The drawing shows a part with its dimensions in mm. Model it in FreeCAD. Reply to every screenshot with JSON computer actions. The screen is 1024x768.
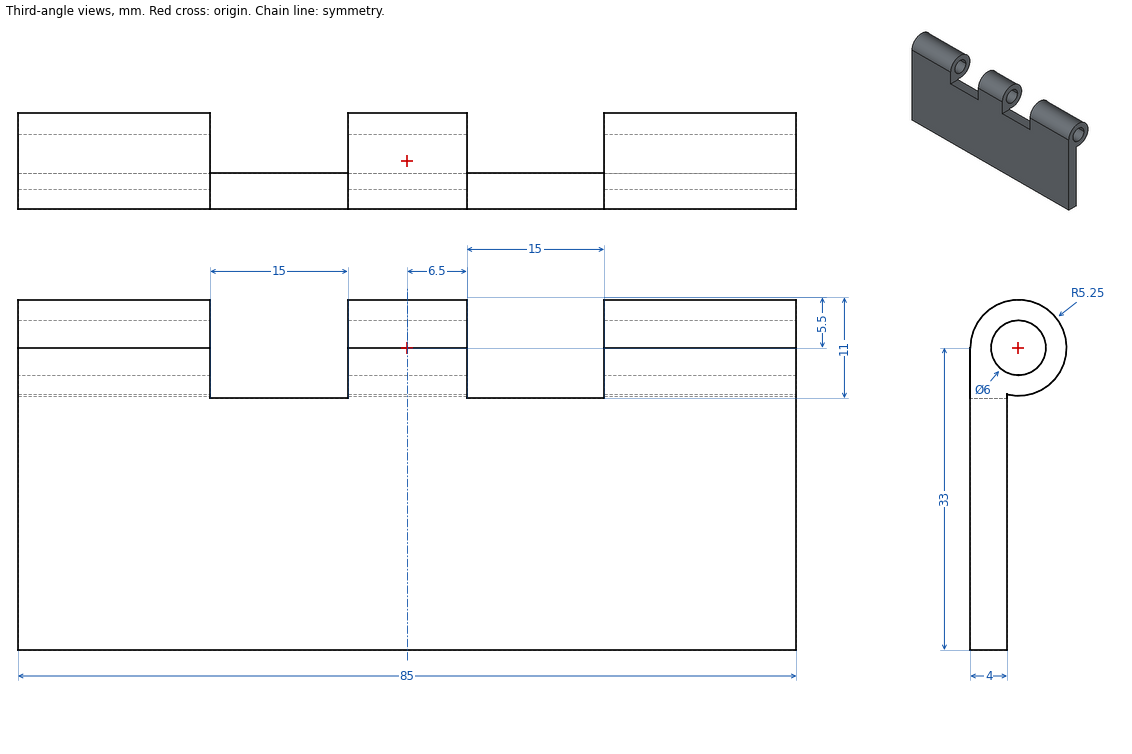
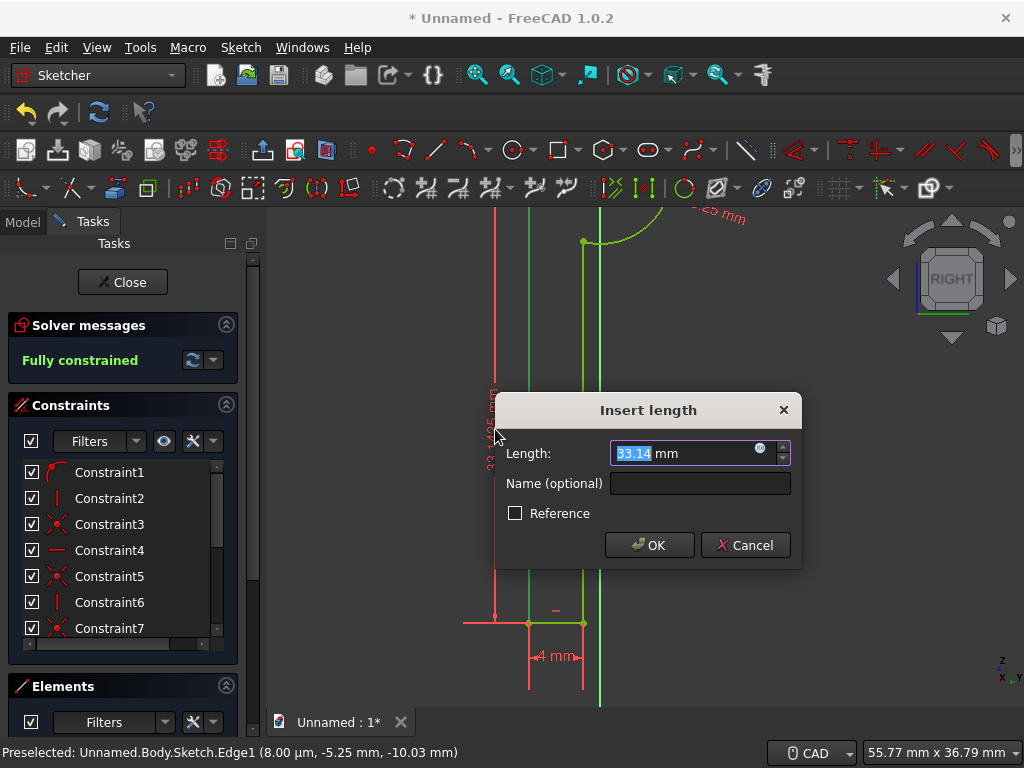
{"action": "type", "text": "33"}
{"action": "key", "text": "Return"}
{"action": "key", "text": "Escape"}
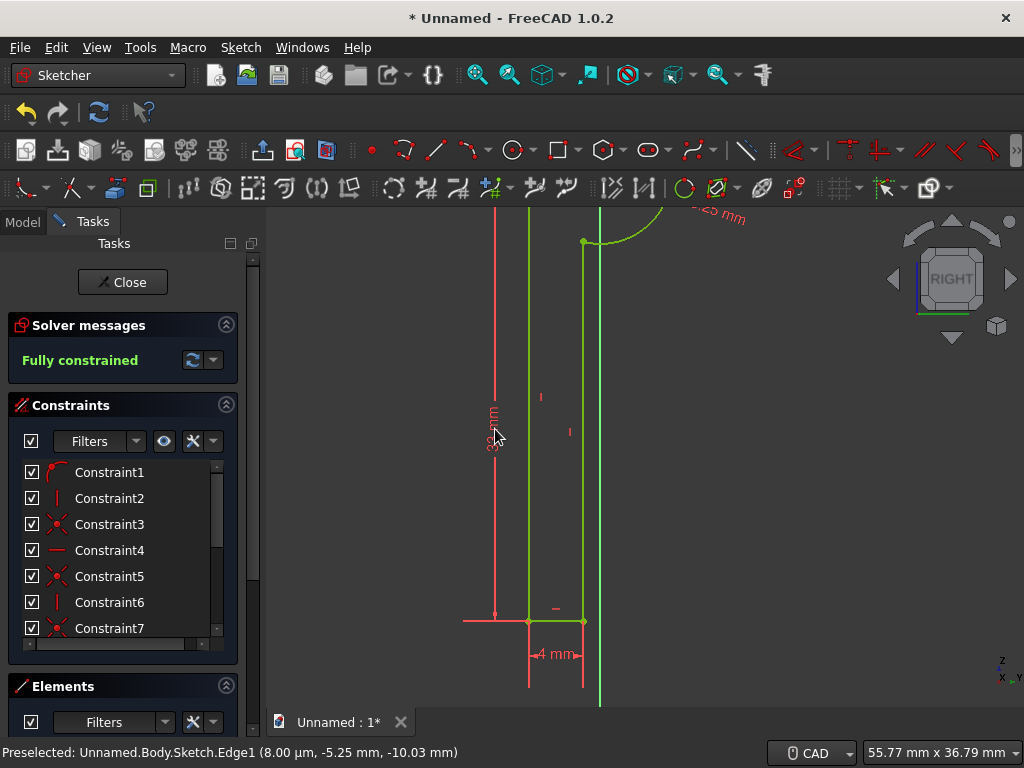
{"action": "left_click", "coordinate": [123, 282]}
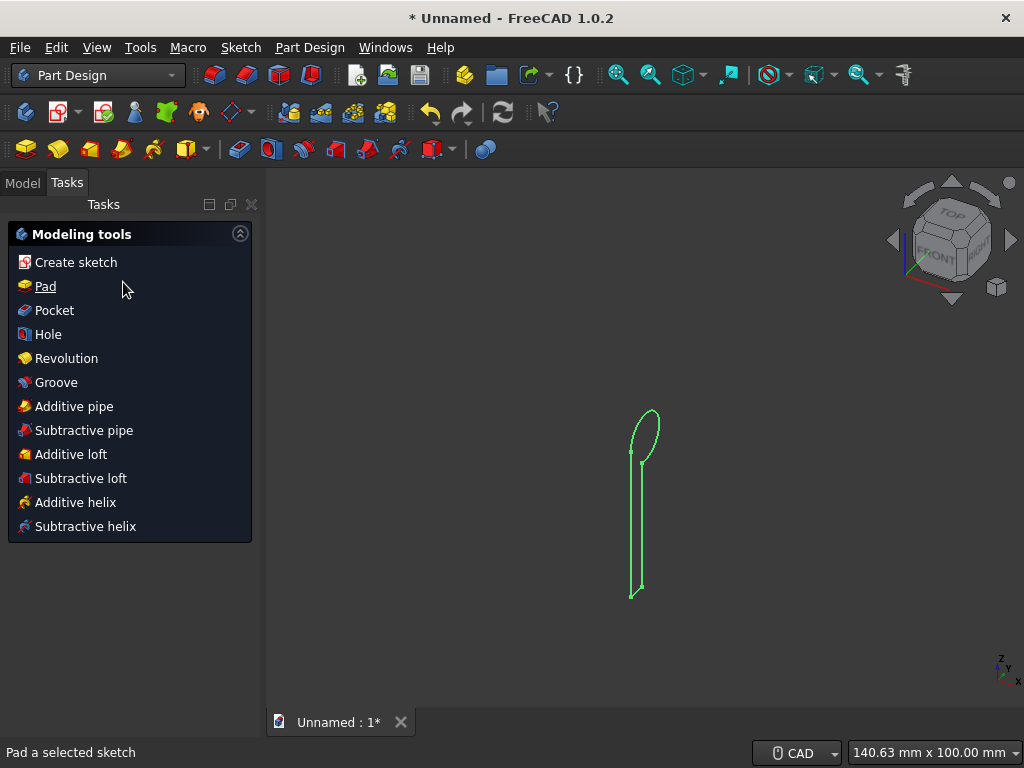
{"action": "left_click", "coordinate": [26, 150]}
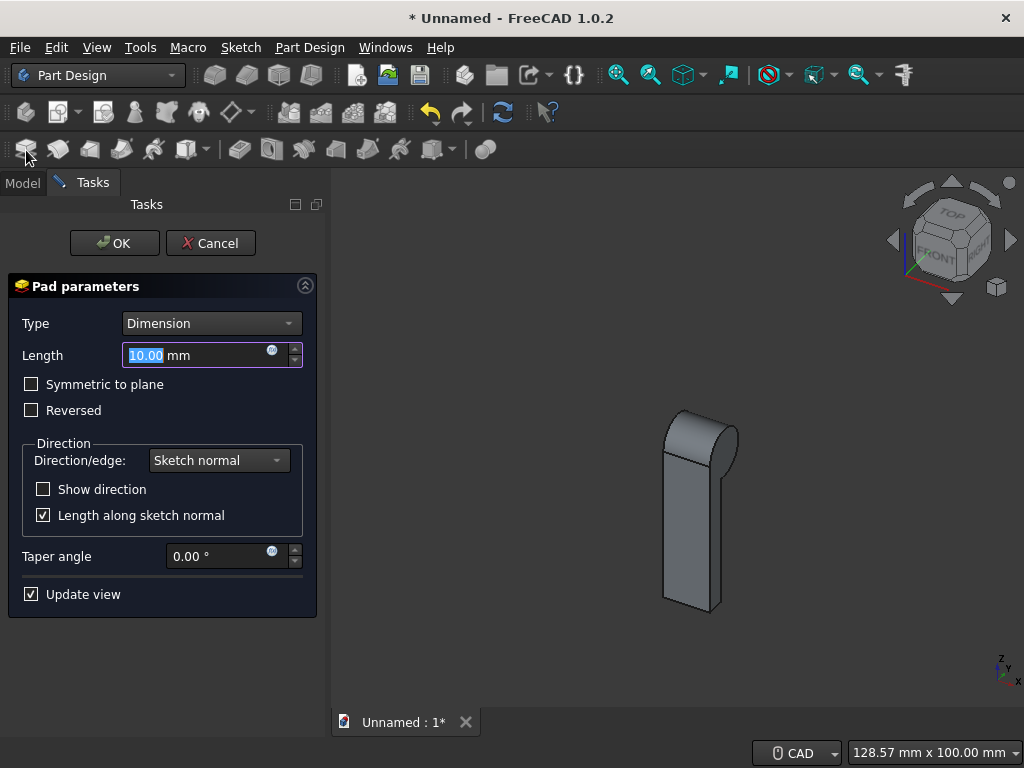
{"action": "type", "text": "85"}
{"action": "key", "text": "Tab"}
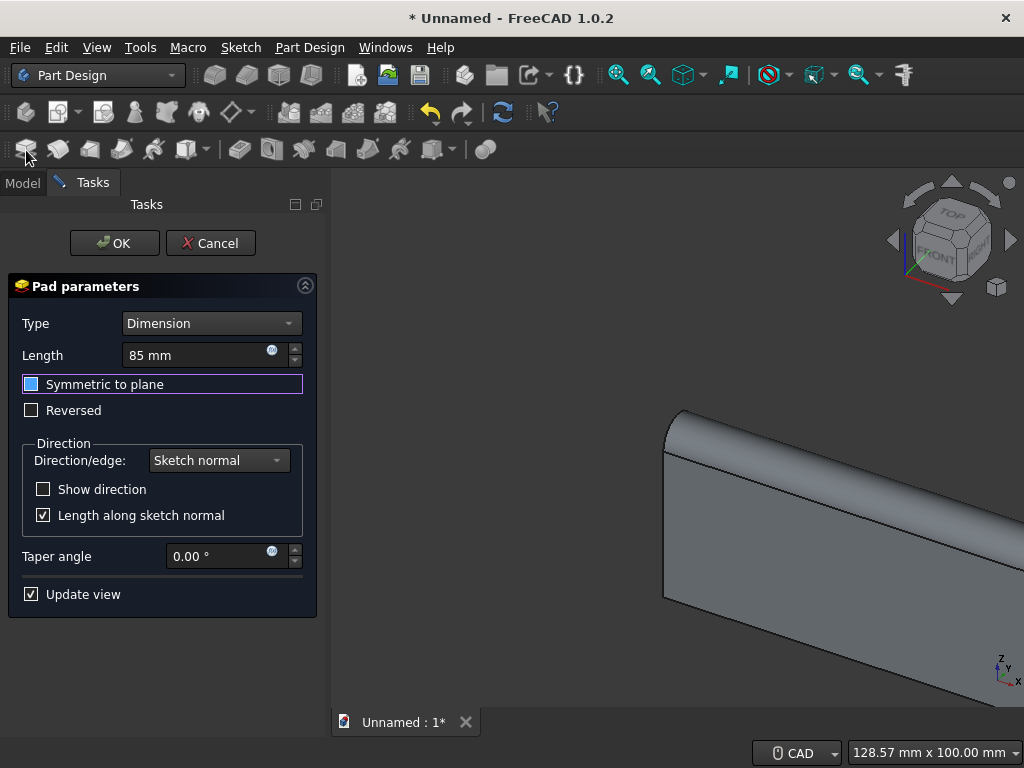
{"action": "left_click", "coordinate": [30, 384]}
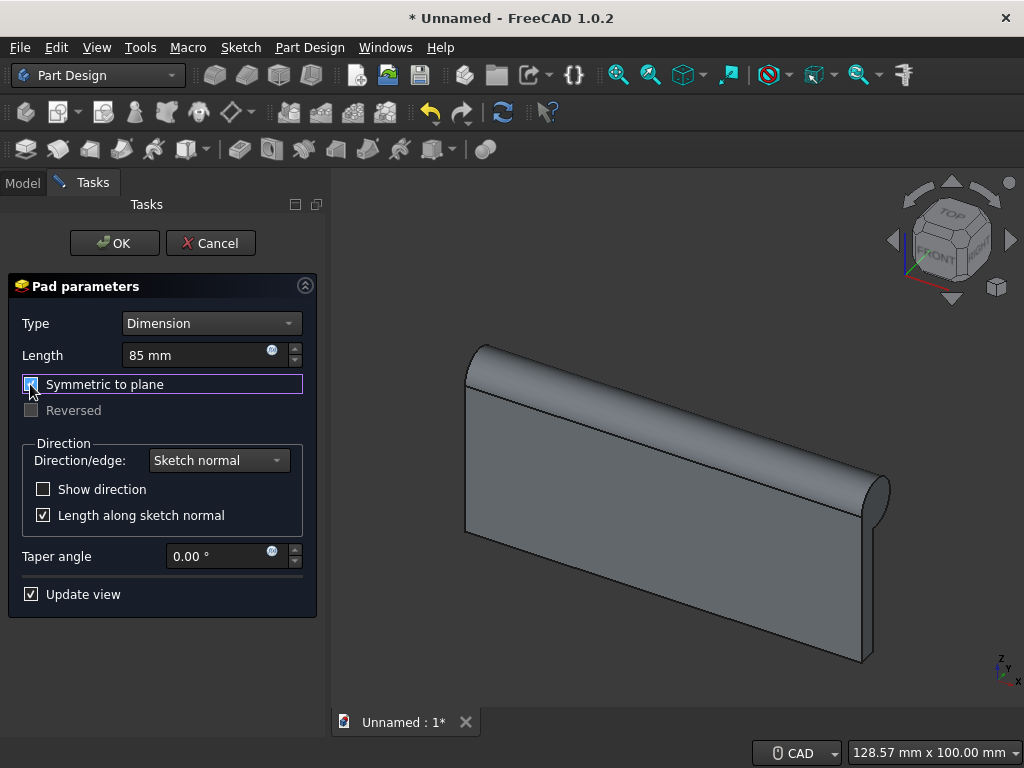
{"action": "left_click", "coordinate": [115, 243]}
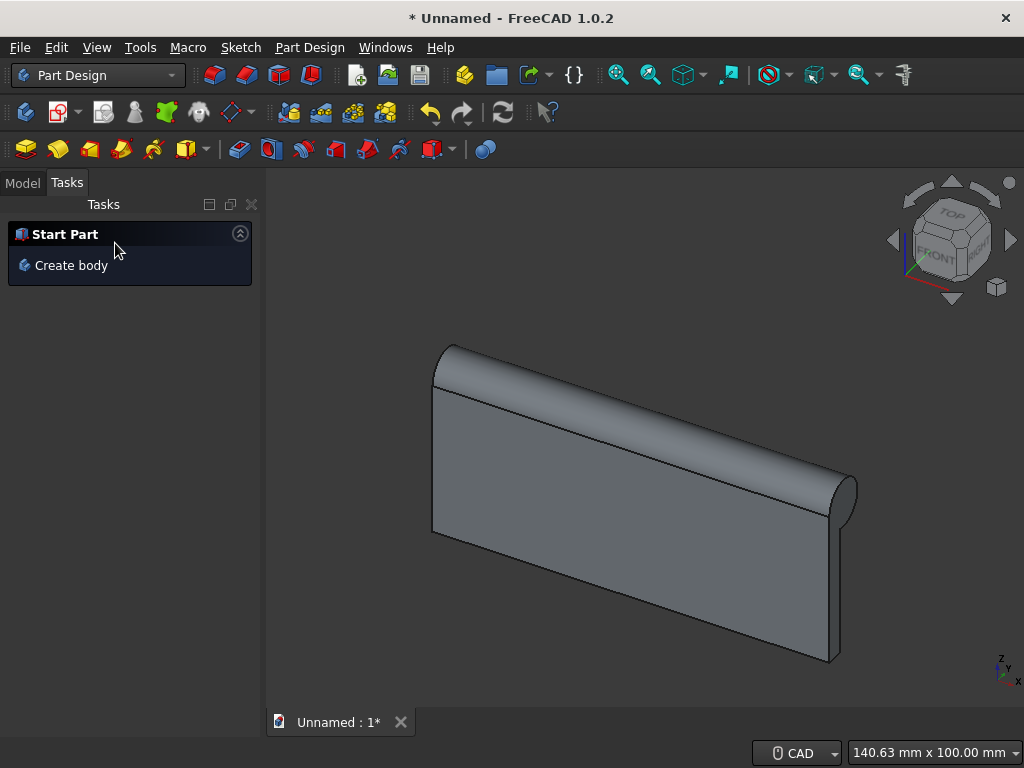
{"action": "left_click", "coordinate": [58, 112]}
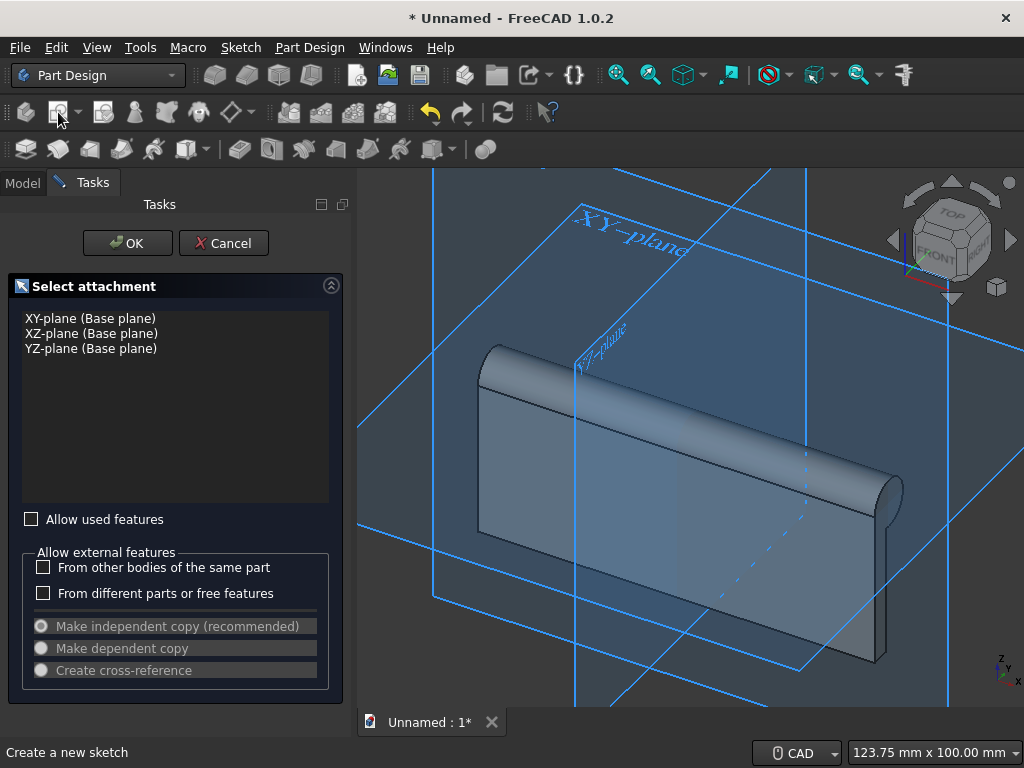
{"action": "left_click", "coordinate": [82, 334]}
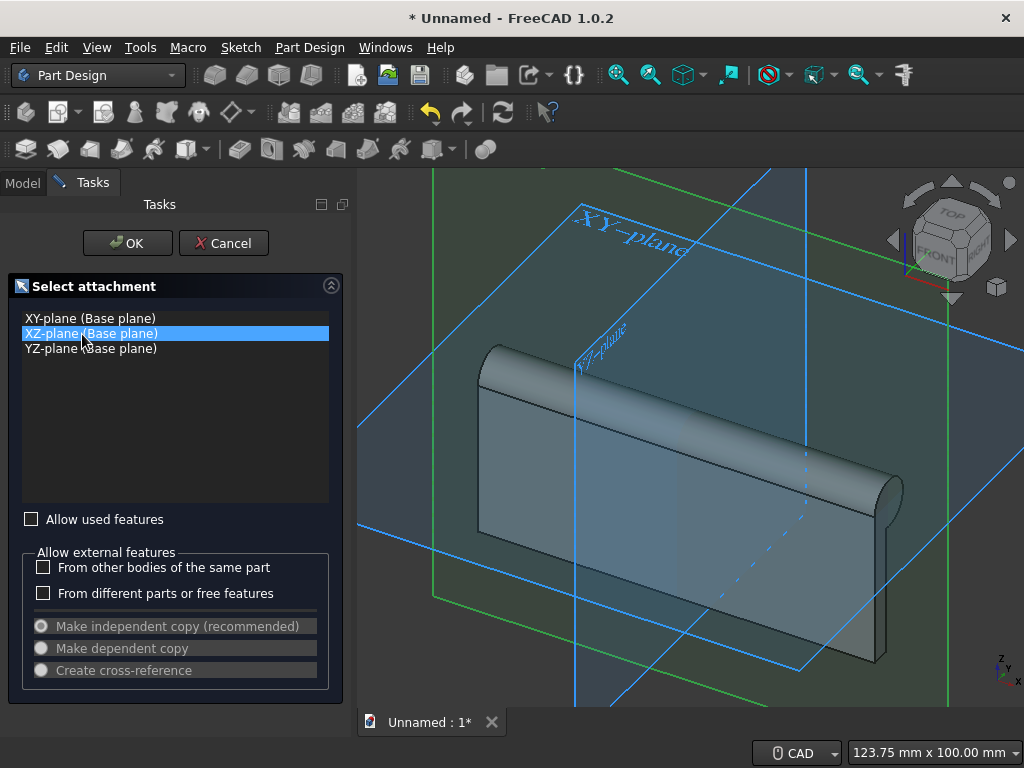
{"action": "left_click", "coordinate": [128, 243]}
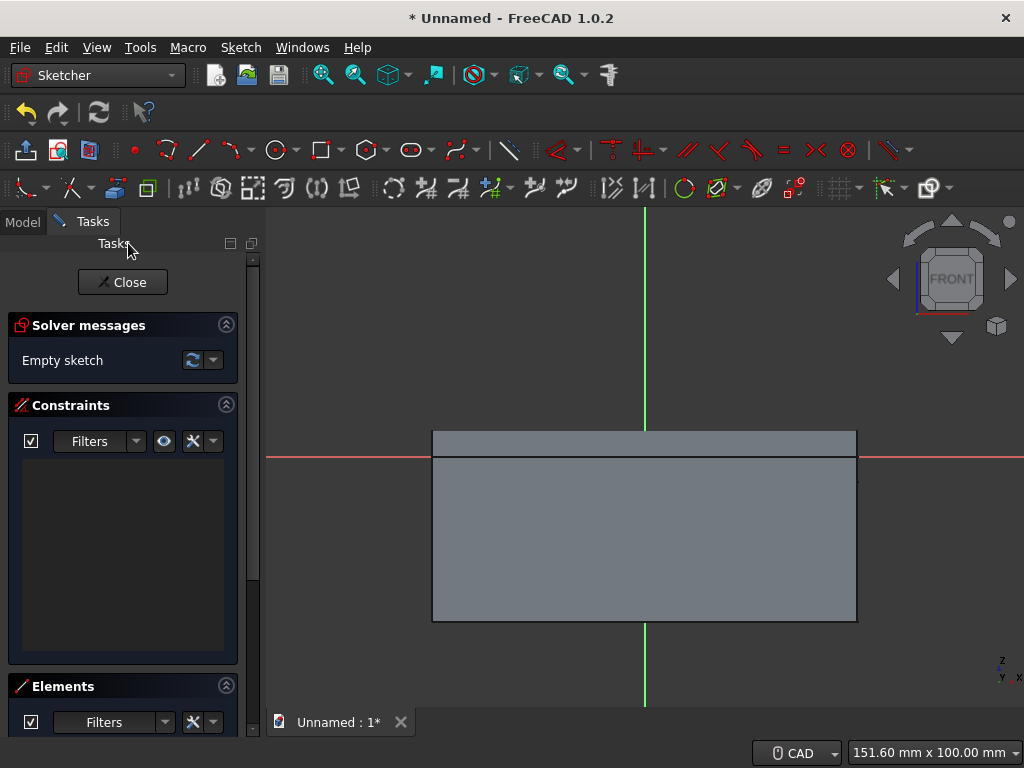
{"action": "left_click", "coordinate": [90, 150]}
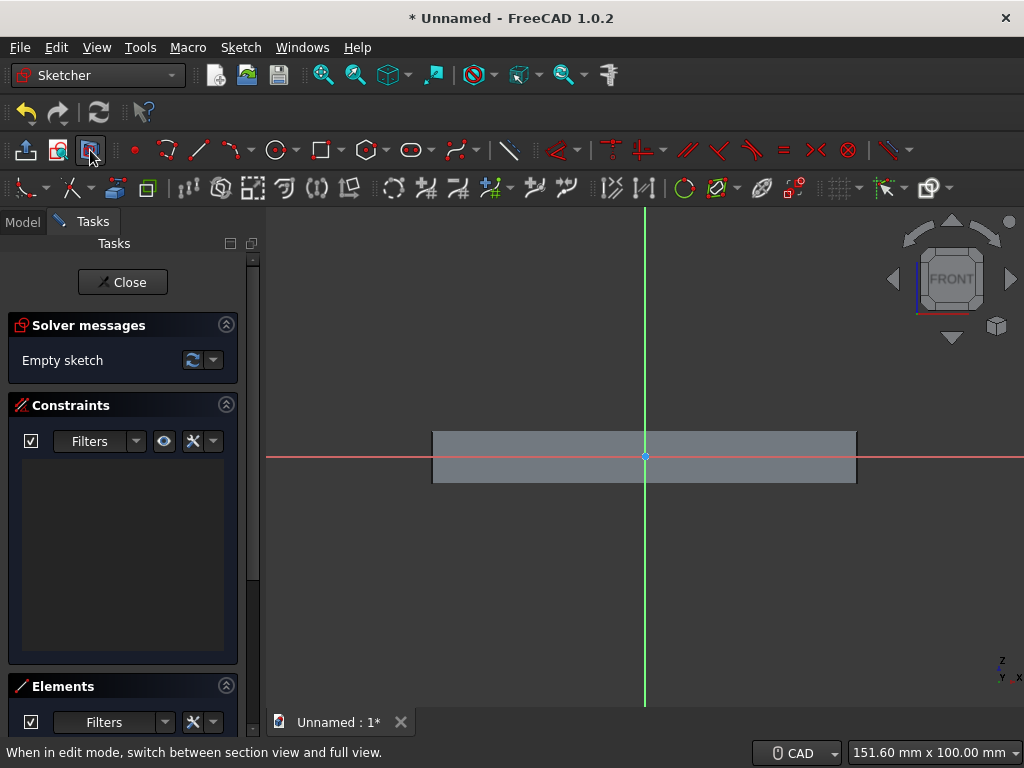
{"action": "scroll", "coordinate": [728, 457], "scroll_direction": "up", "scroll_amount": 3}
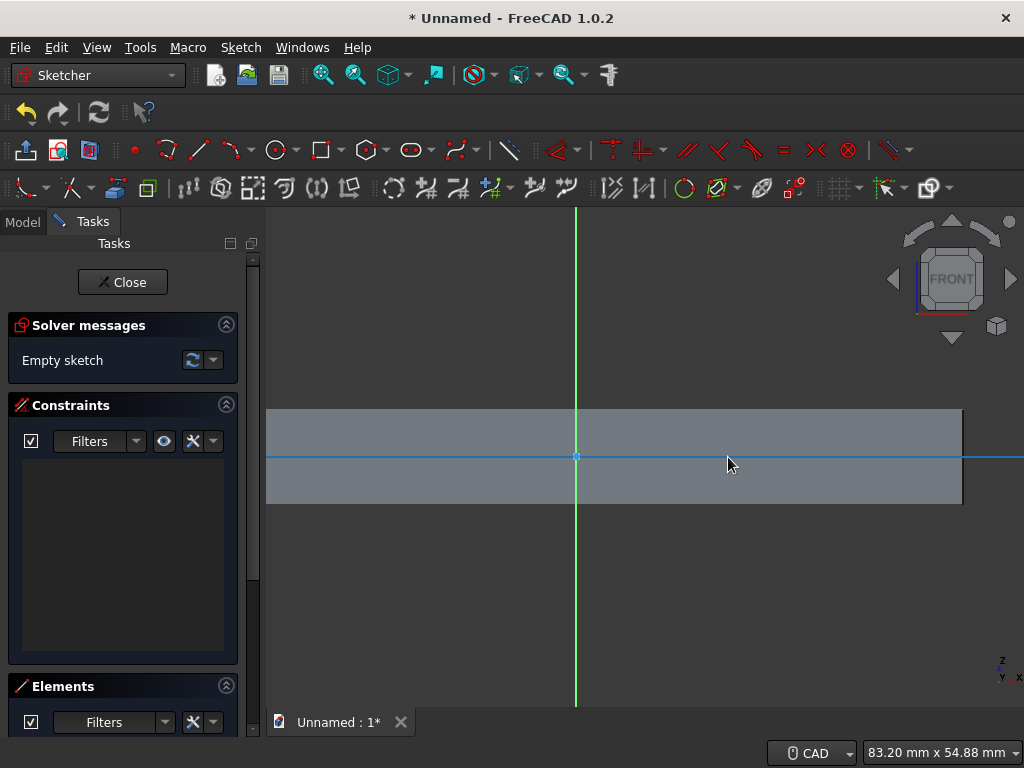
{"action": "left_click", "coordinate": [322, 150]}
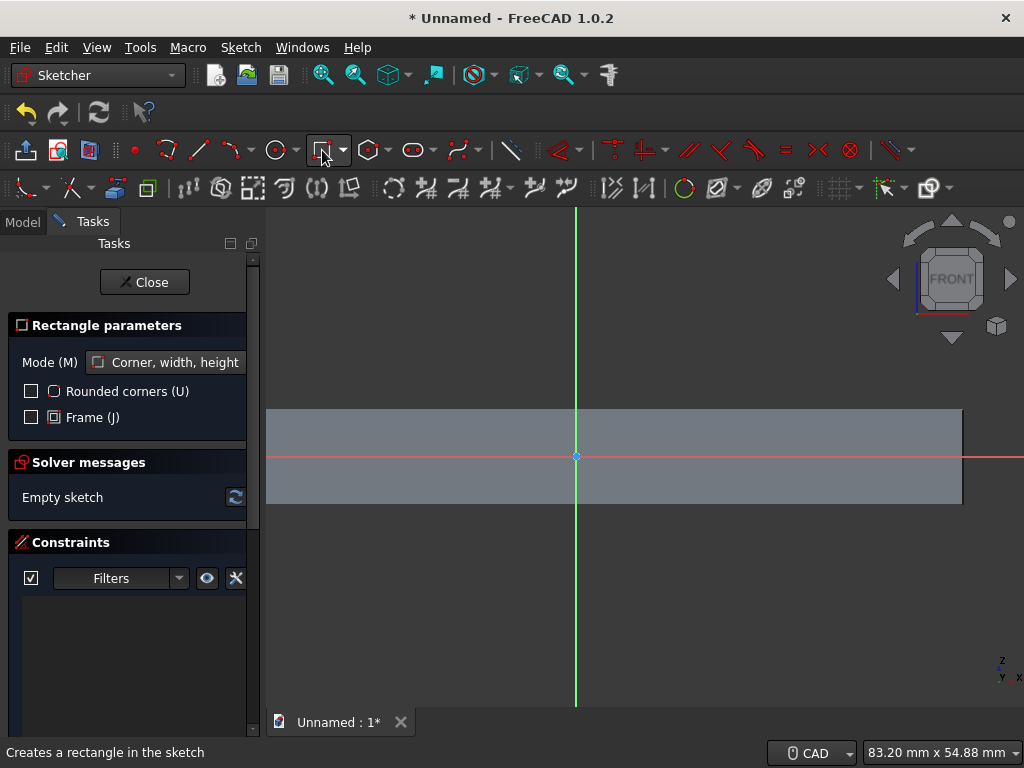
{"action": "left_click", "coordinate": [635, 406]}
{"action": "mouse_move", "coordinate": [772, 507]}